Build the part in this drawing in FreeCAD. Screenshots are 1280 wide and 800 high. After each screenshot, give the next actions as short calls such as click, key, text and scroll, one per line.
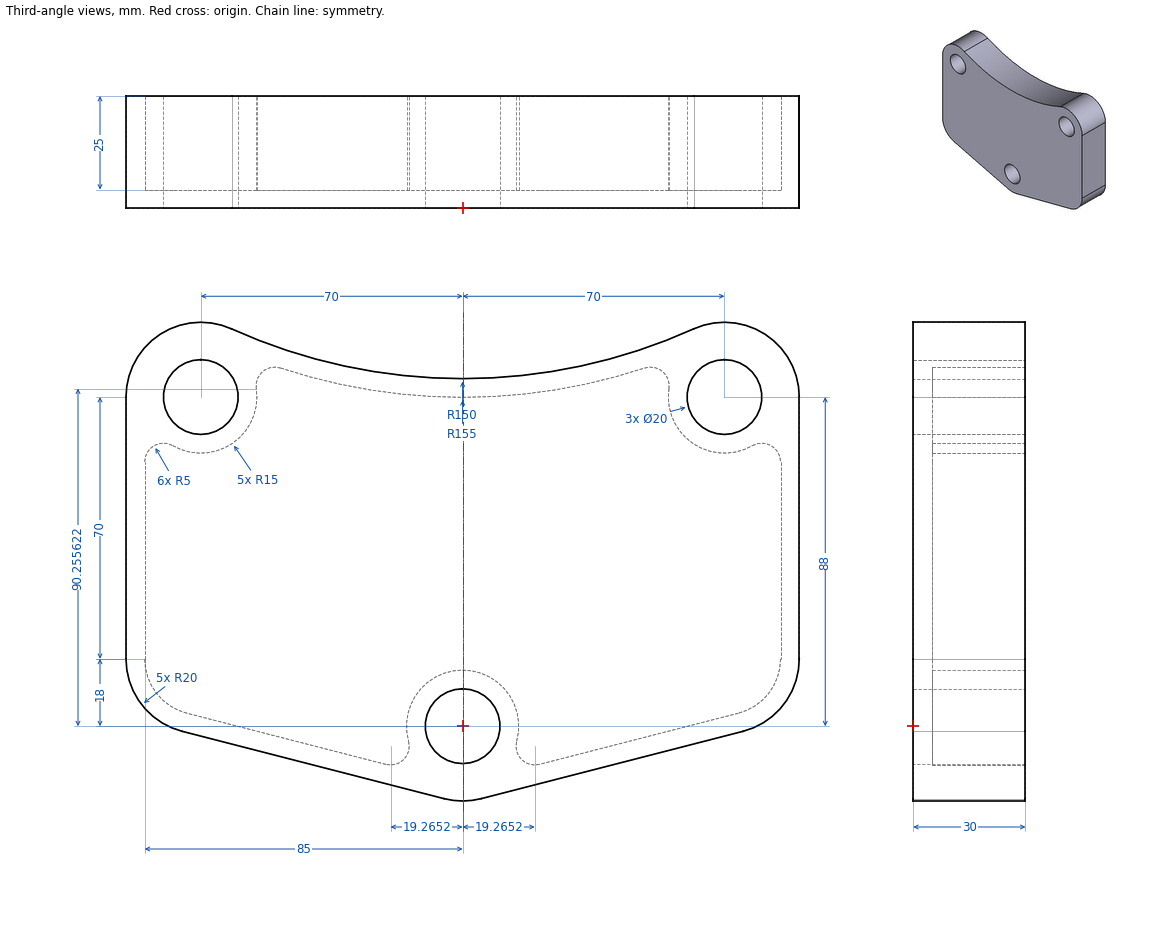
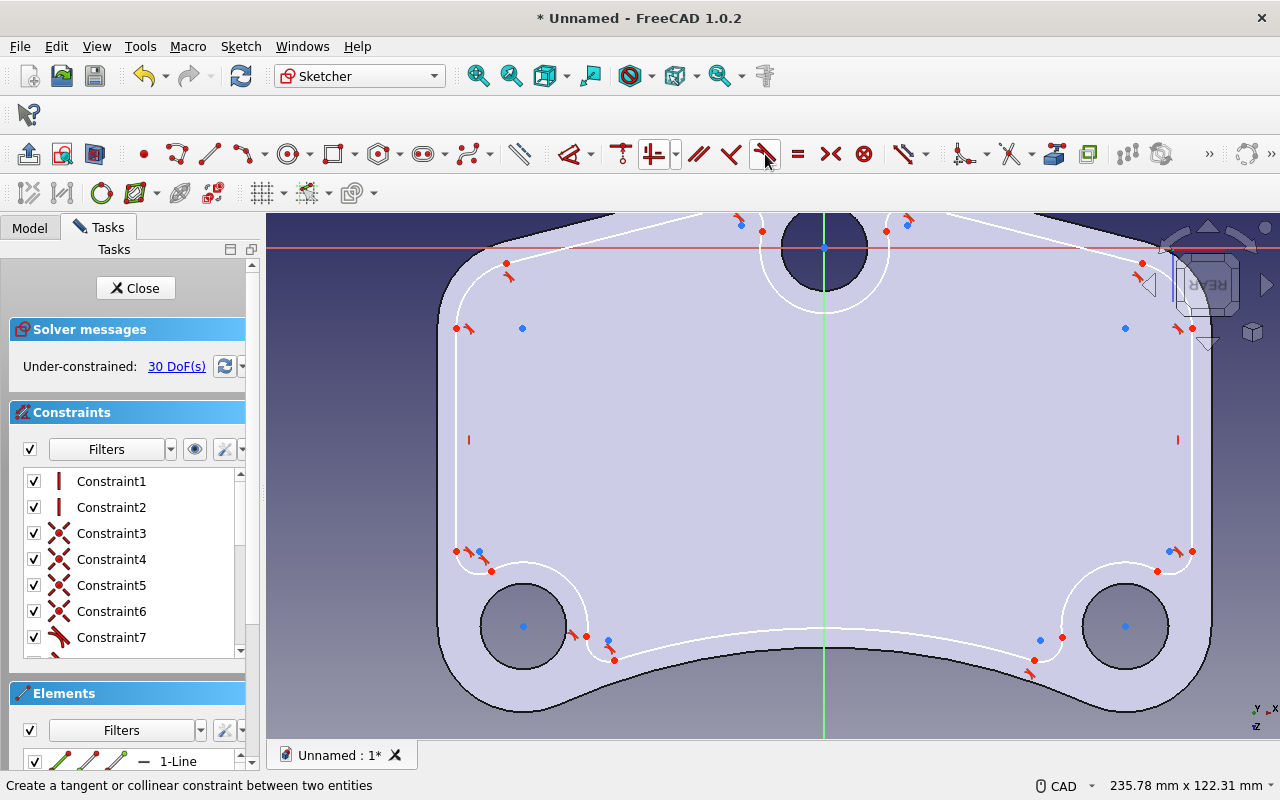
click(1047, 661)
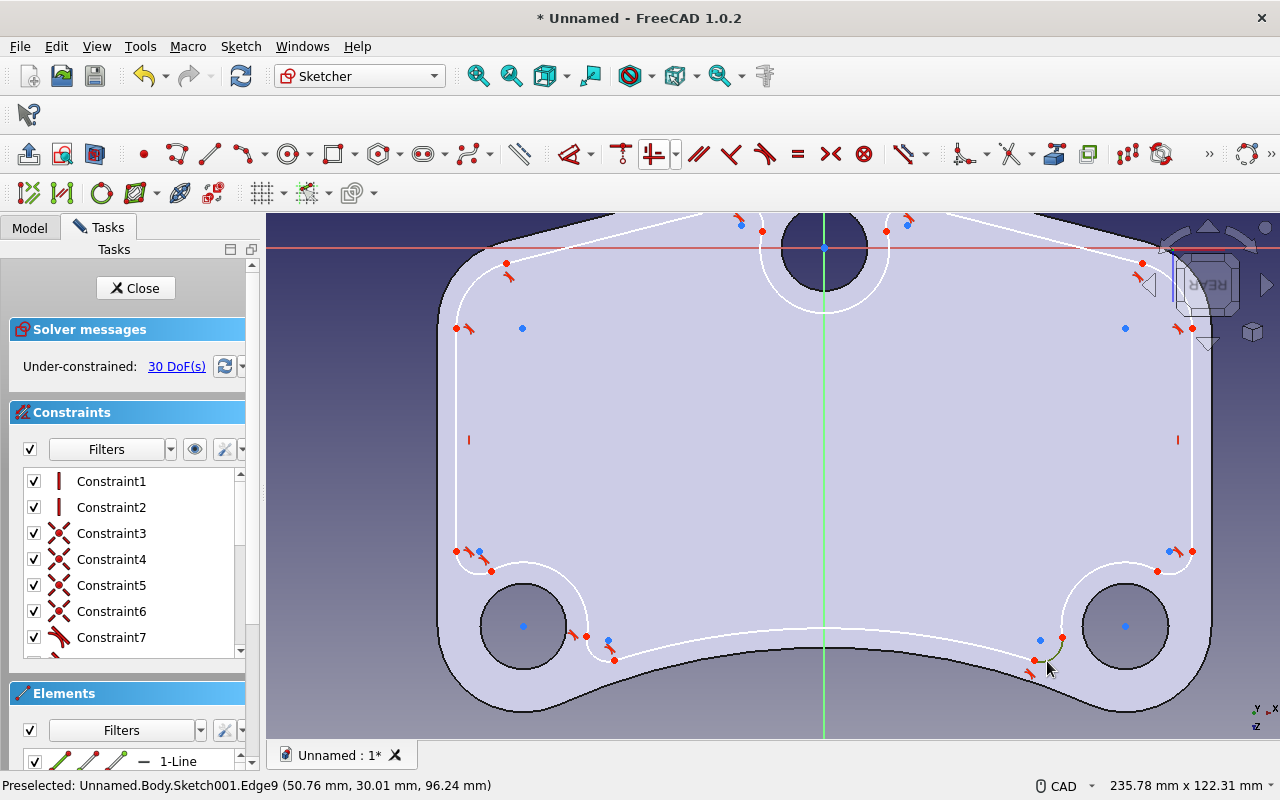
click(1070, 595)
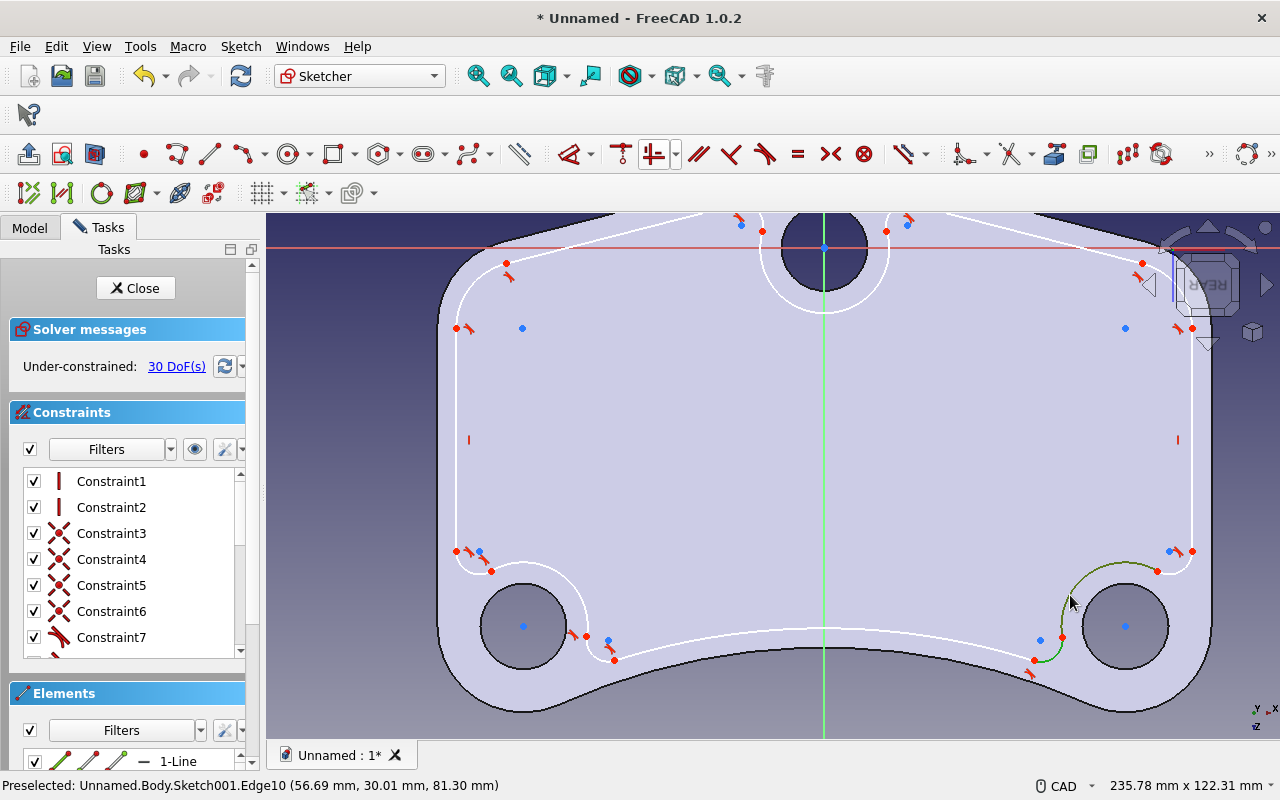
click(765, 154)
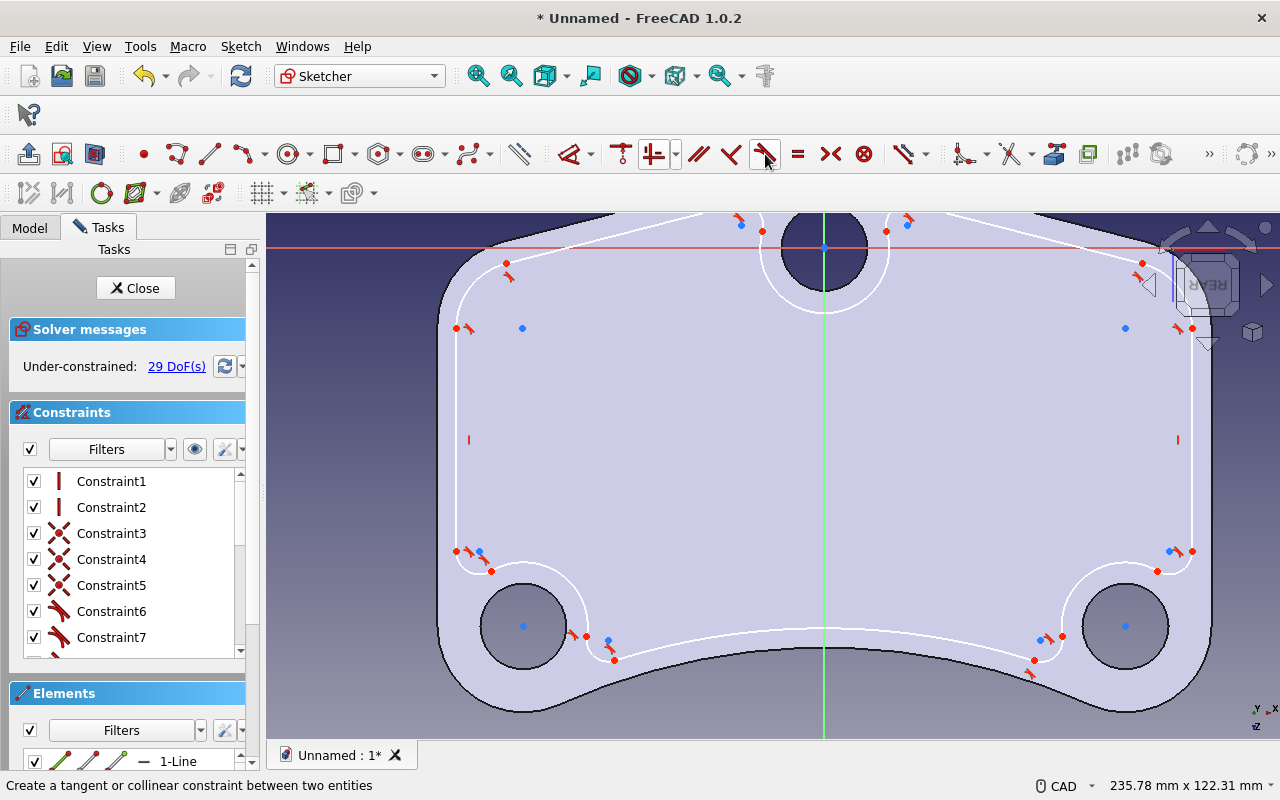
click(1070, 595)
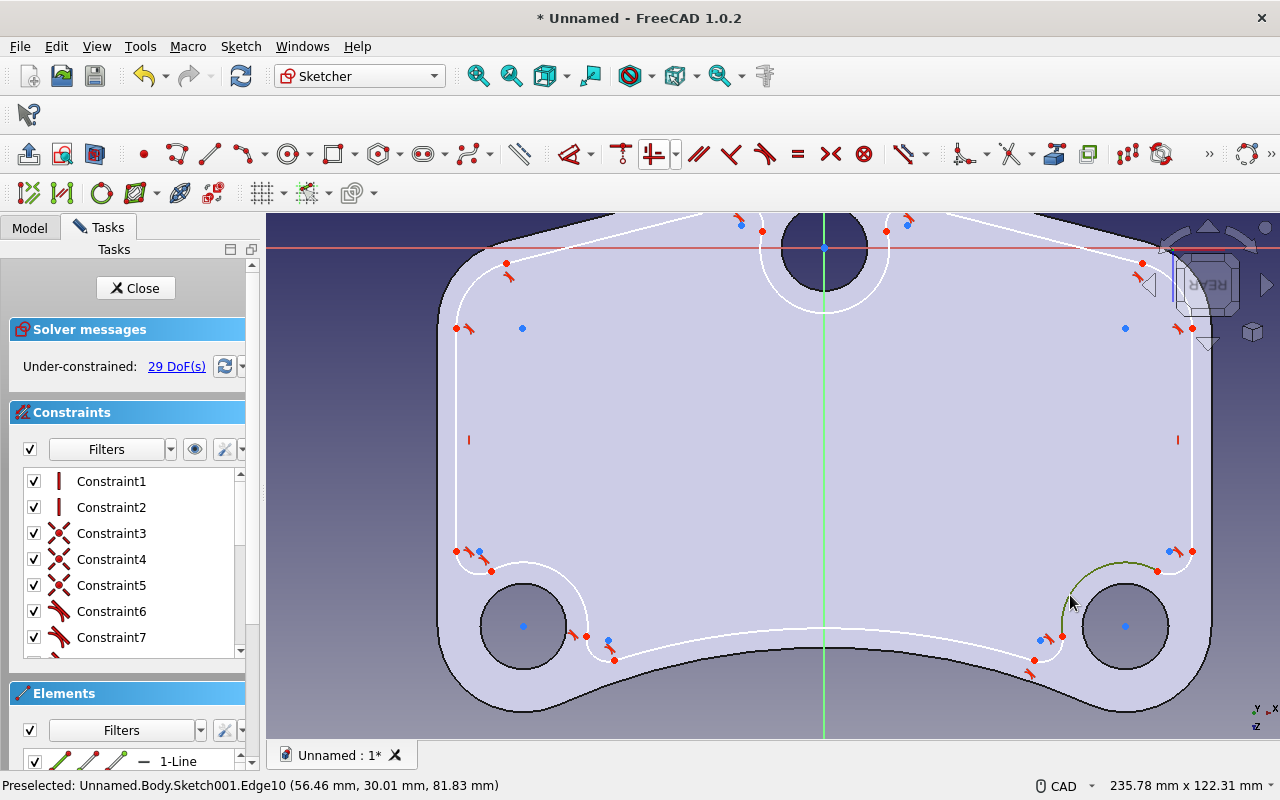
scroll(461, 566, down, 2)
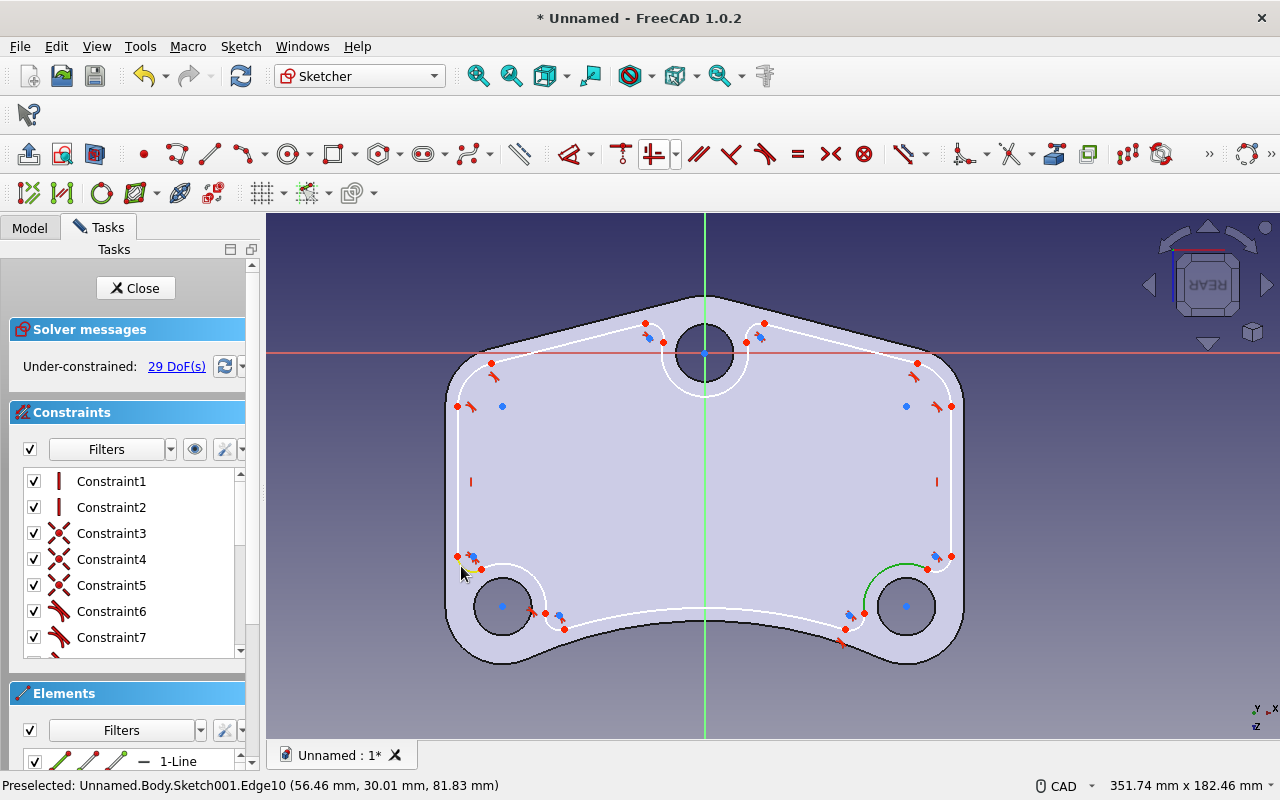
scroll(937, 572, up, 2)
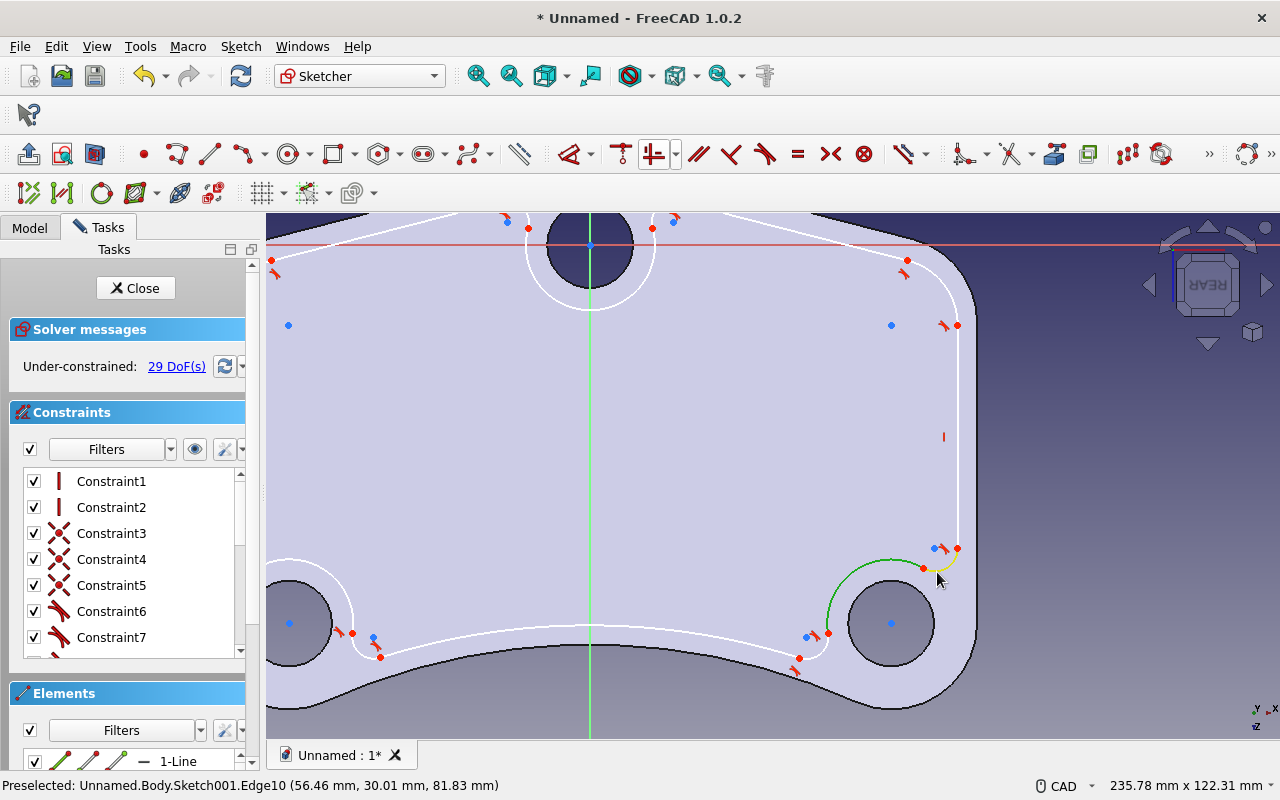
click(937, 571)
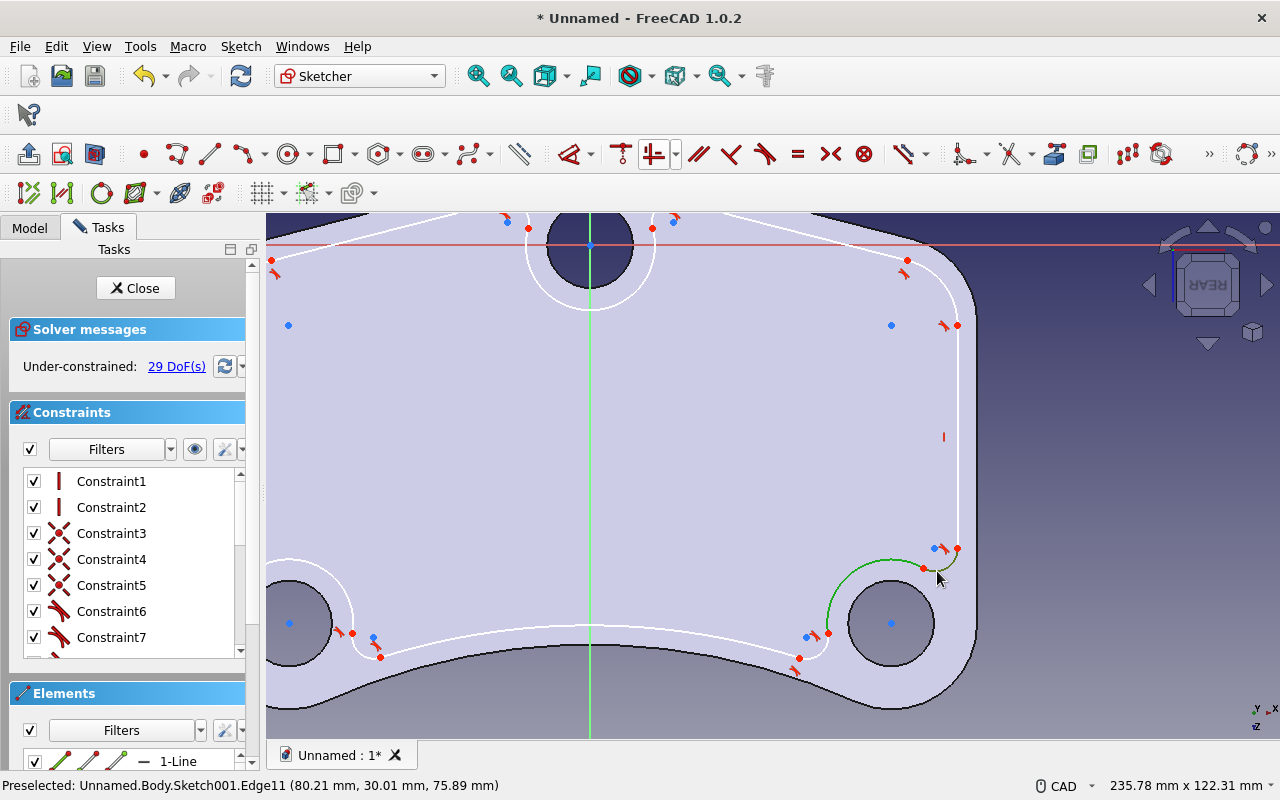
click(765, 154)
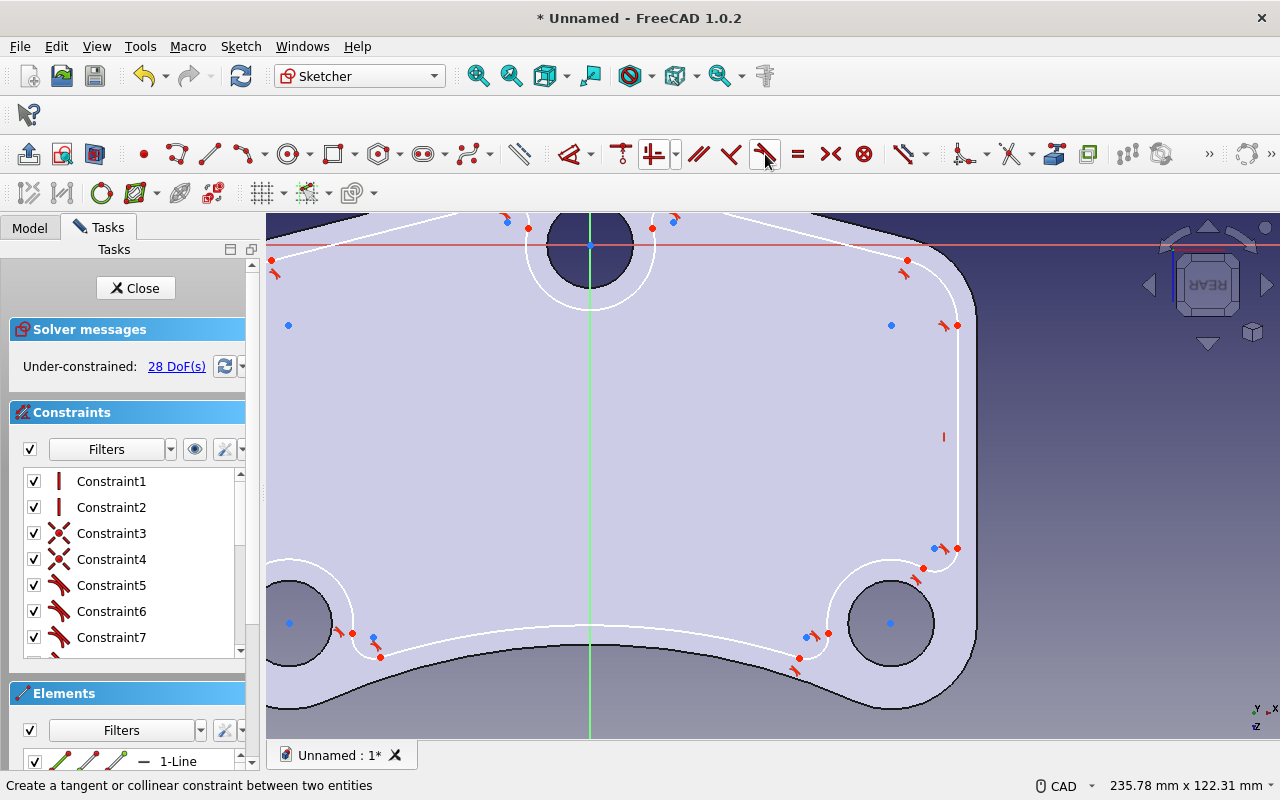
scroll(937, 572, down, 2)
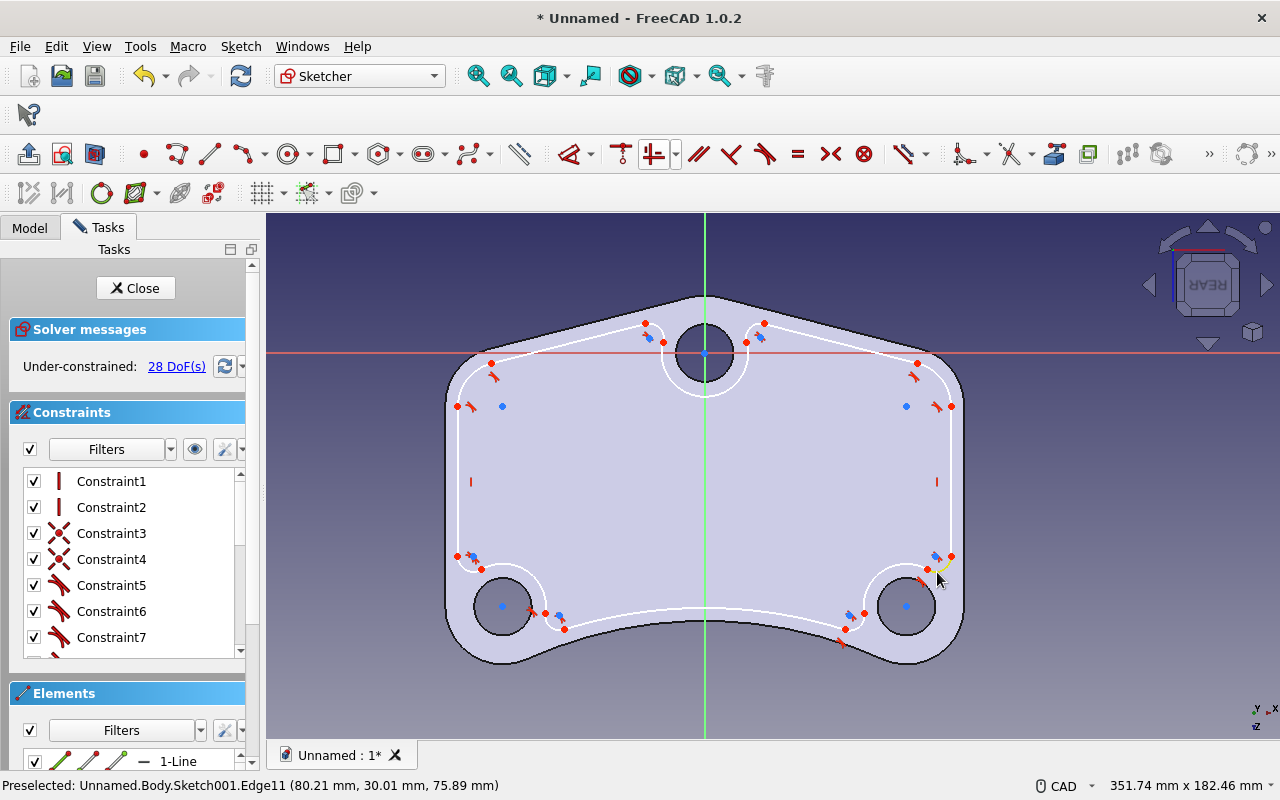
scroll(755, 325, up, 3)